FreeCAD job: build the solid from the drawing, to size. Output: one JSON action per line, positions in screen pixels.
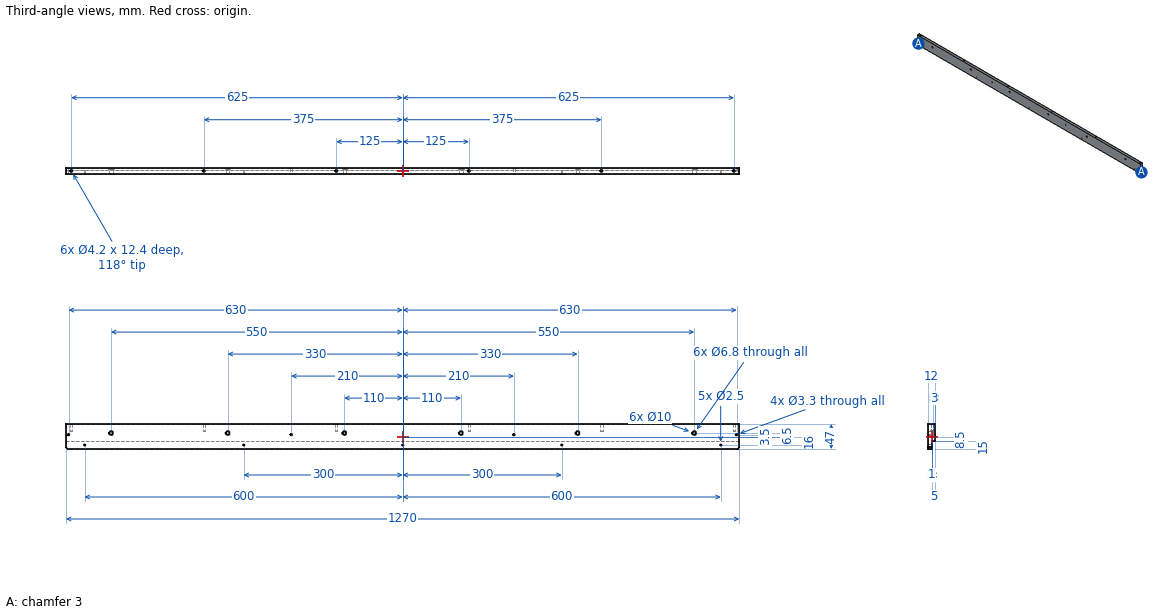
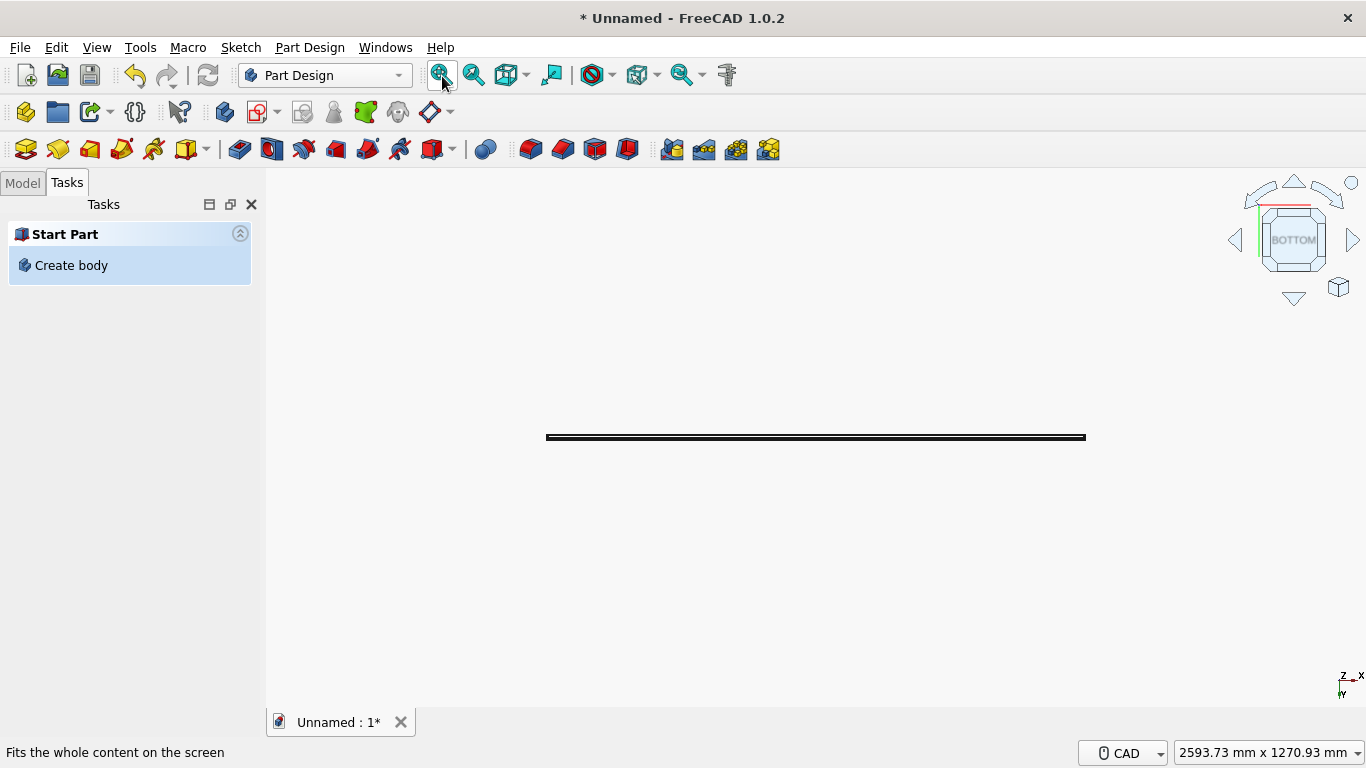
{"action": "key", "text": "0"}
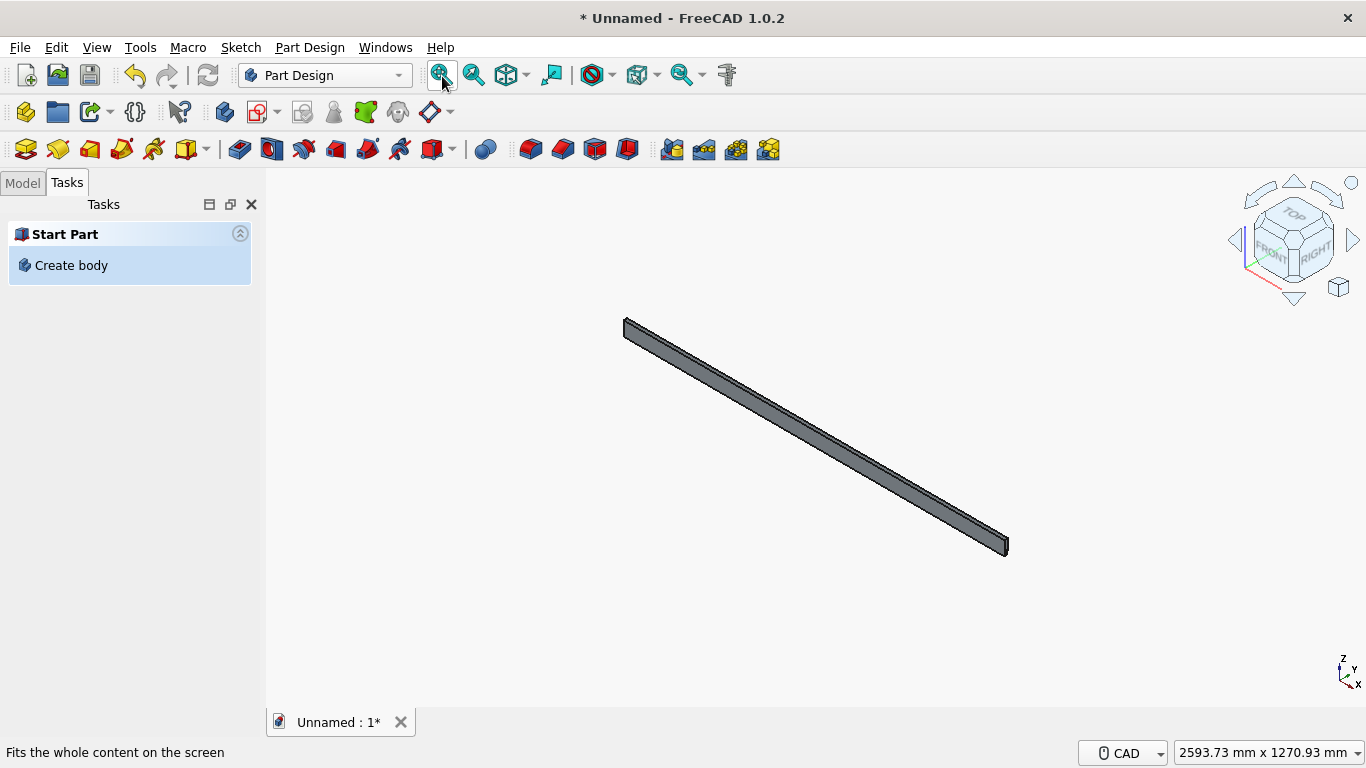
{"action": "left_click", "coordinate": [442, 76]}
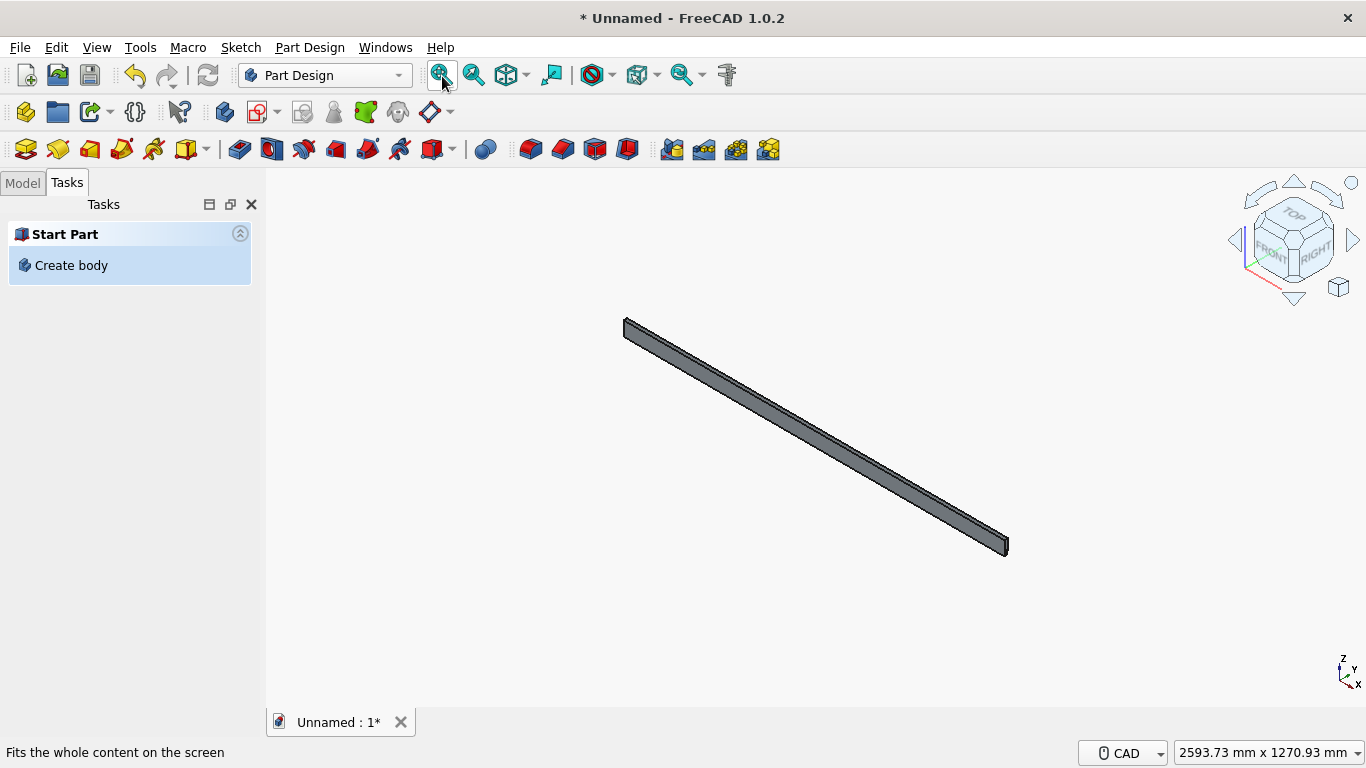
{"action": "scroll", "coordinate": [979, 523], "scroll_direction": "up", "scroll_amount": 8}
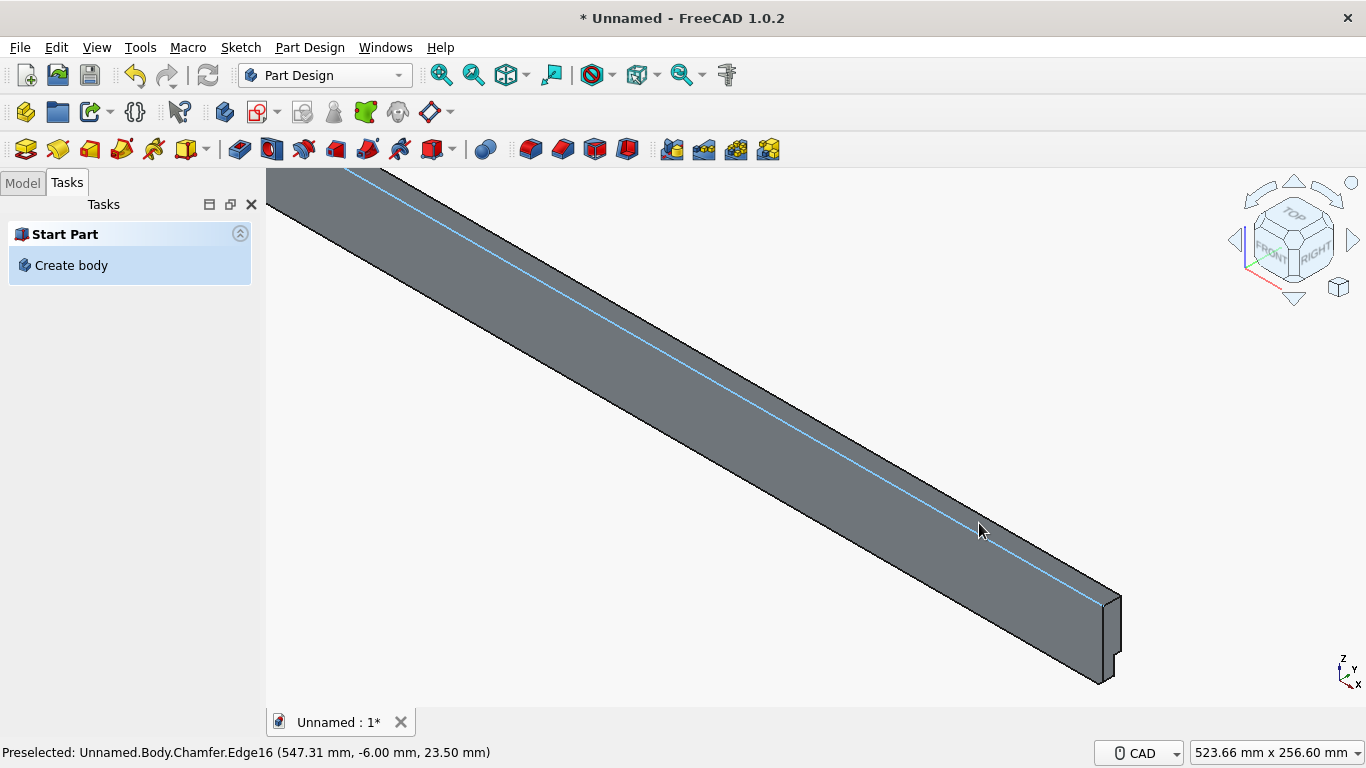
{"action": "left_click", "coordinate": [978, 522]}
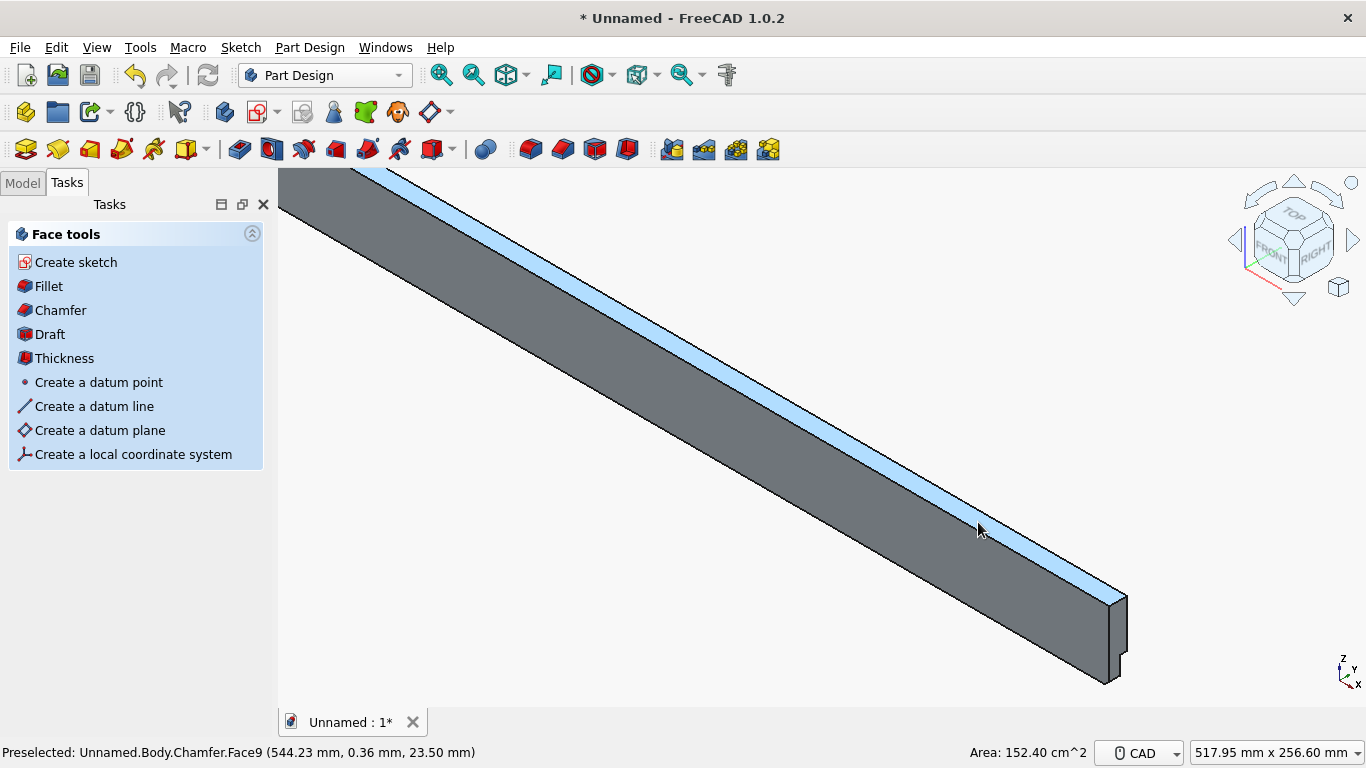
{"action": "left_click", "coordinate": [258, 112]}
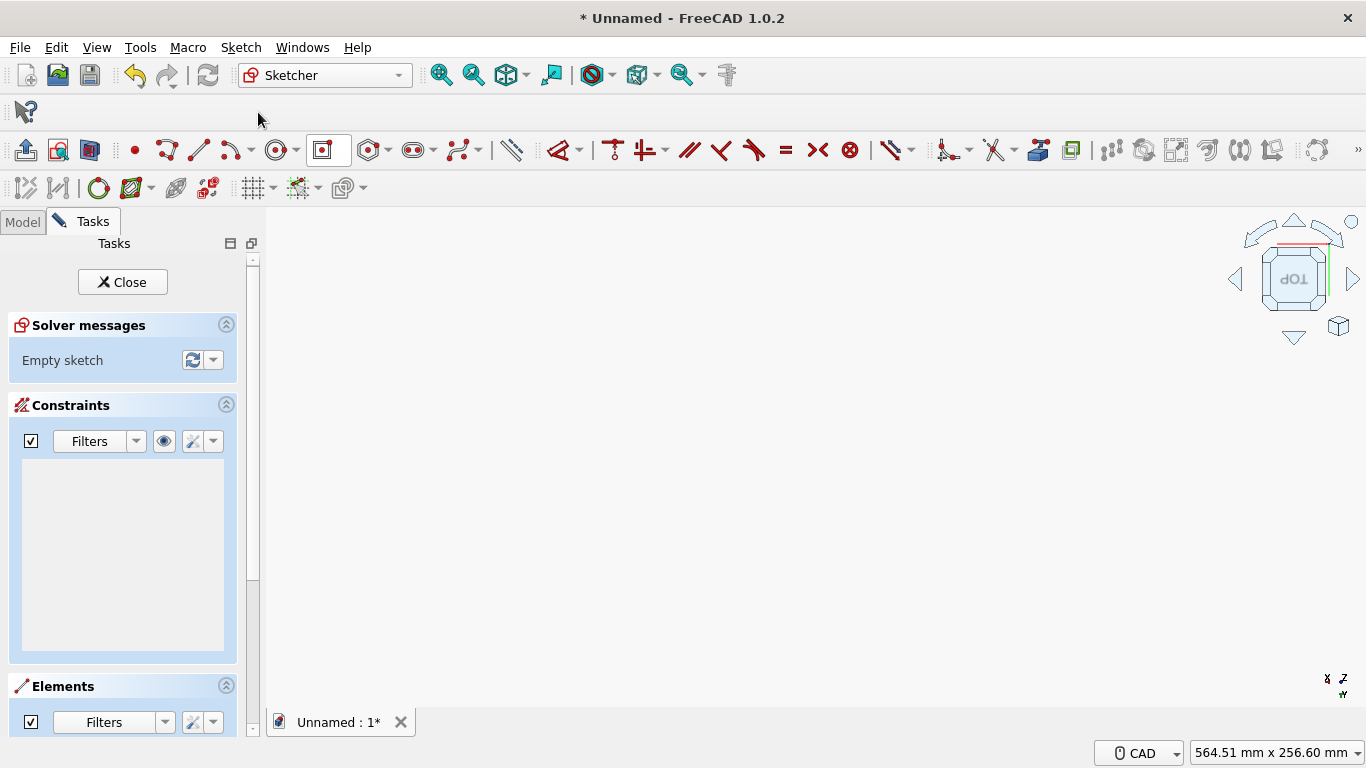
{"action": "scroll", "coordinate": [544, 554], "scroll_direction": "down", "scroll_amount": 7}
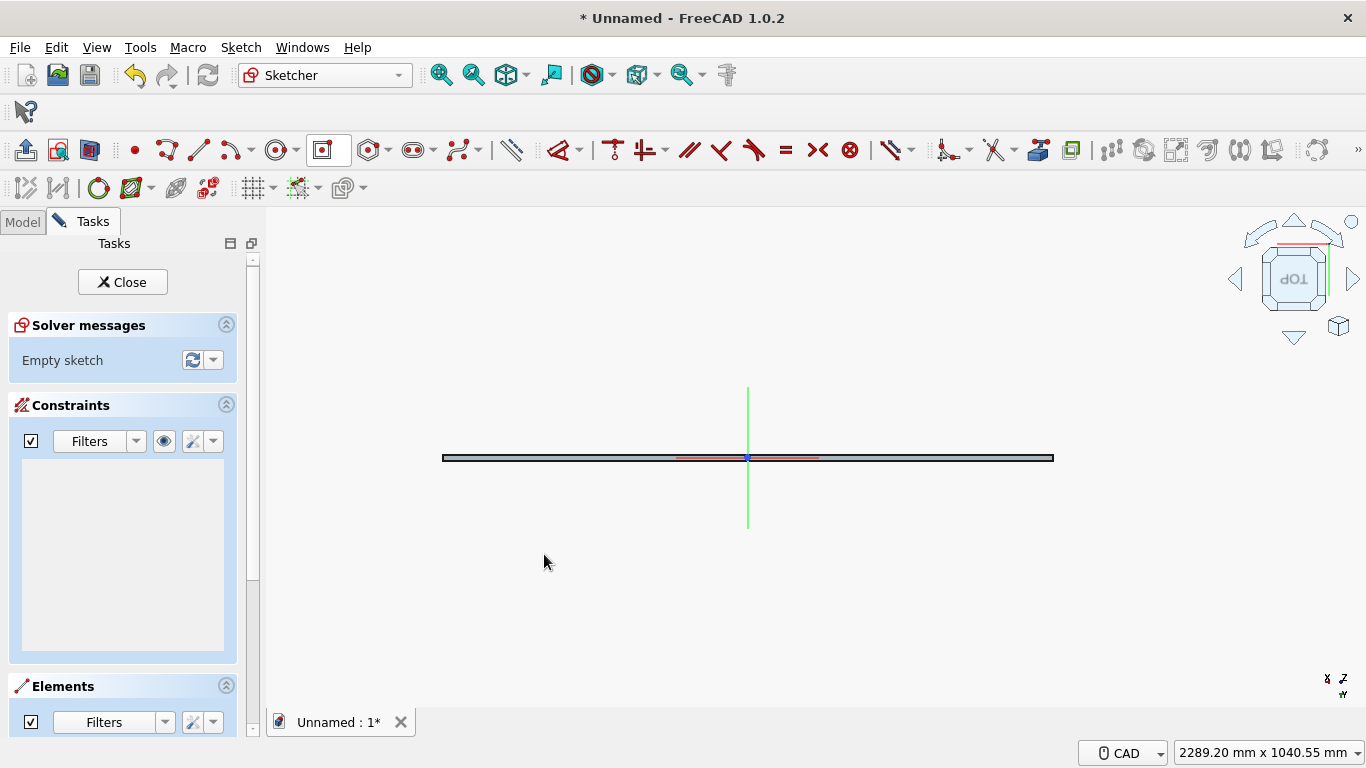
{"action": "key", "text": "g c"}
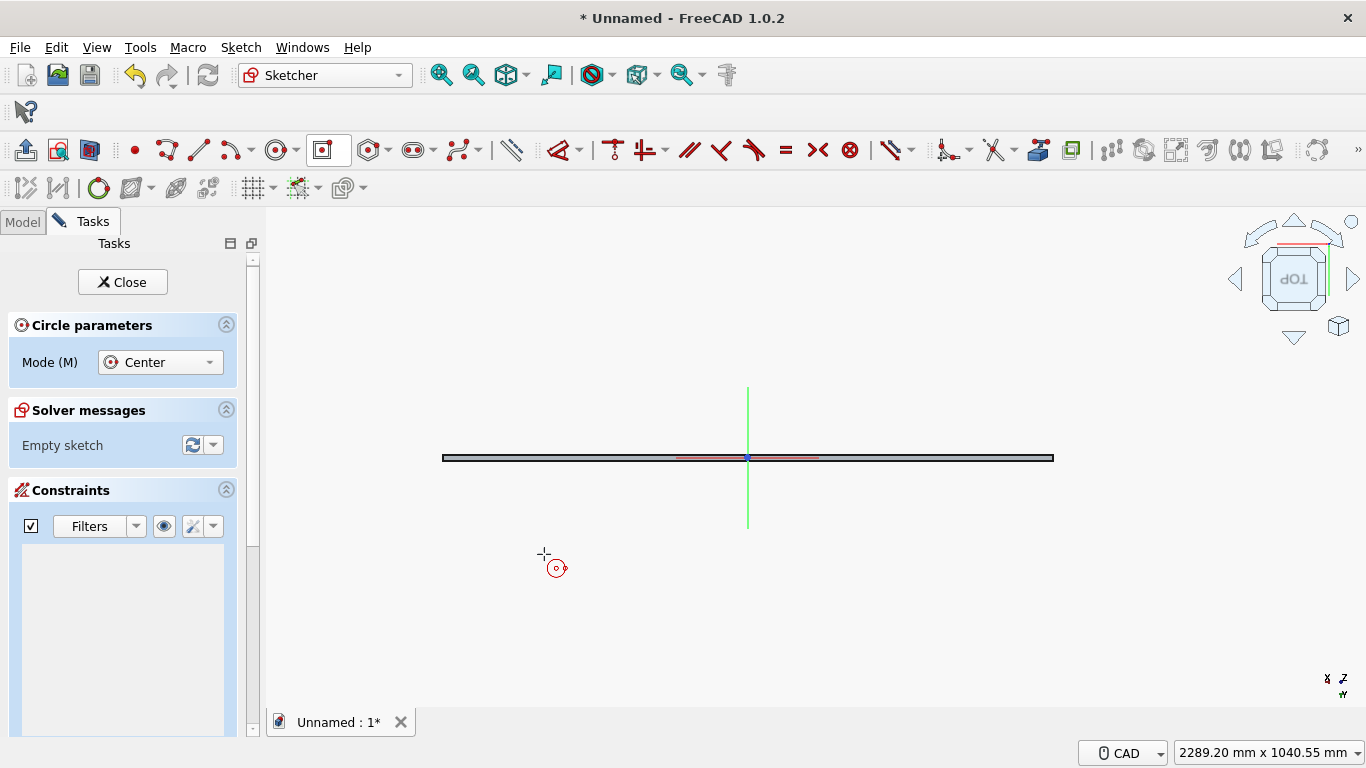
{"action": "scroll", "coordinate": [1048, 458], "scroll_direction": "up", "scroll_amount": 16}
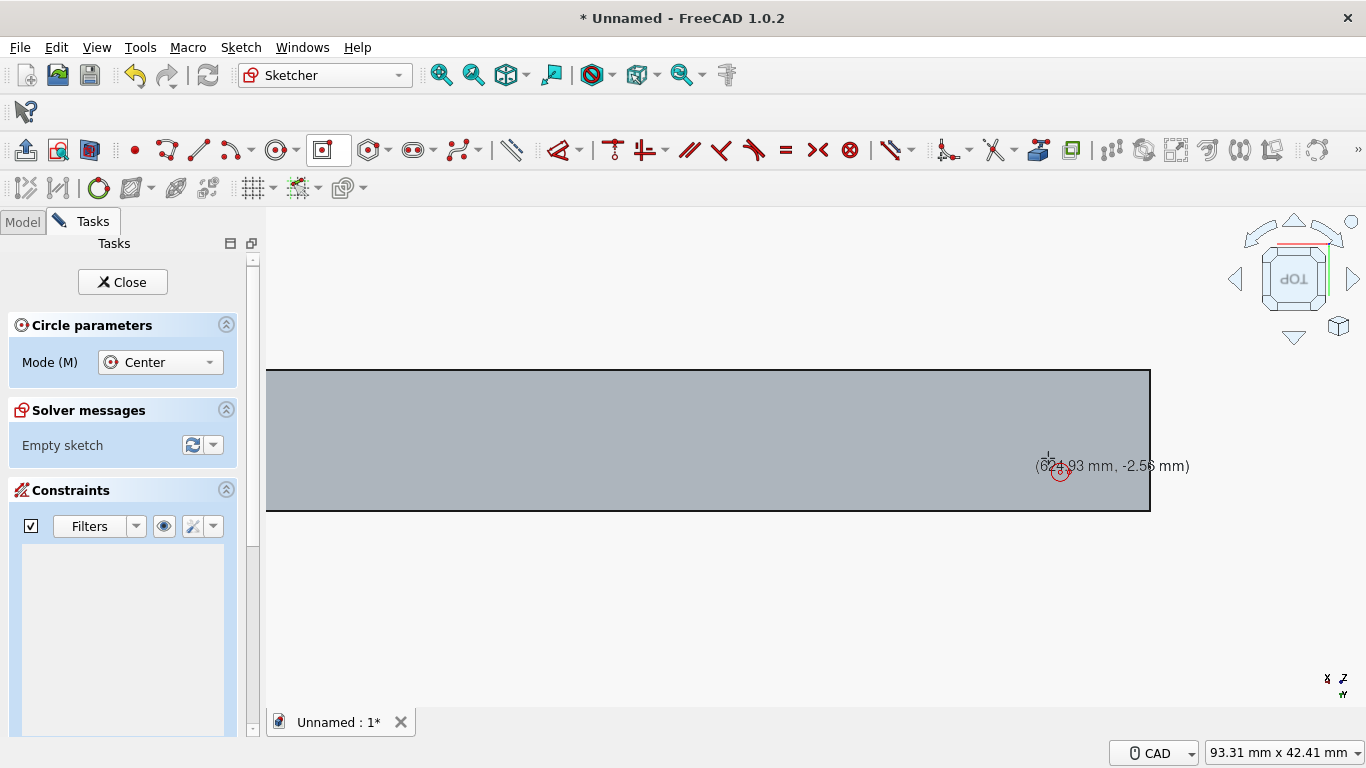
{"action": "scroll", "coordinate": [1119, 458], "scroll_direction": "down", "scroll_amount": 15}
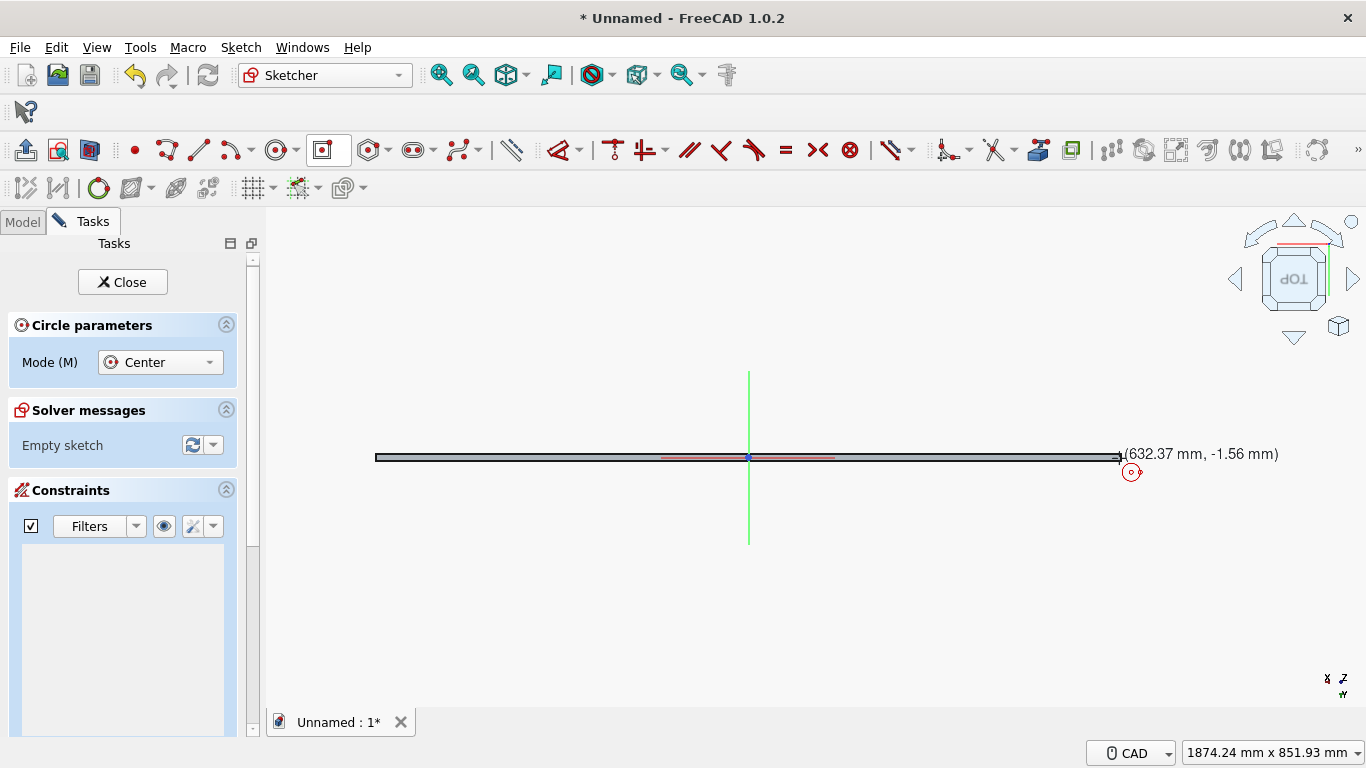
{"action": "left_click", "coordinate": [1115, 458]}